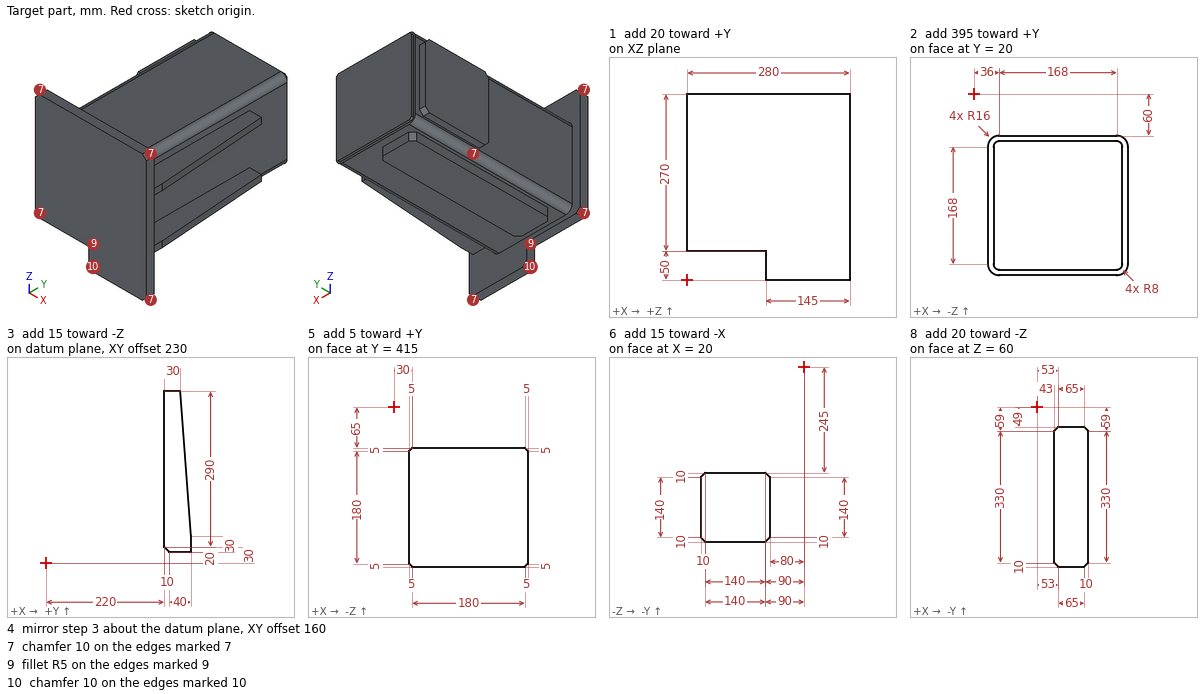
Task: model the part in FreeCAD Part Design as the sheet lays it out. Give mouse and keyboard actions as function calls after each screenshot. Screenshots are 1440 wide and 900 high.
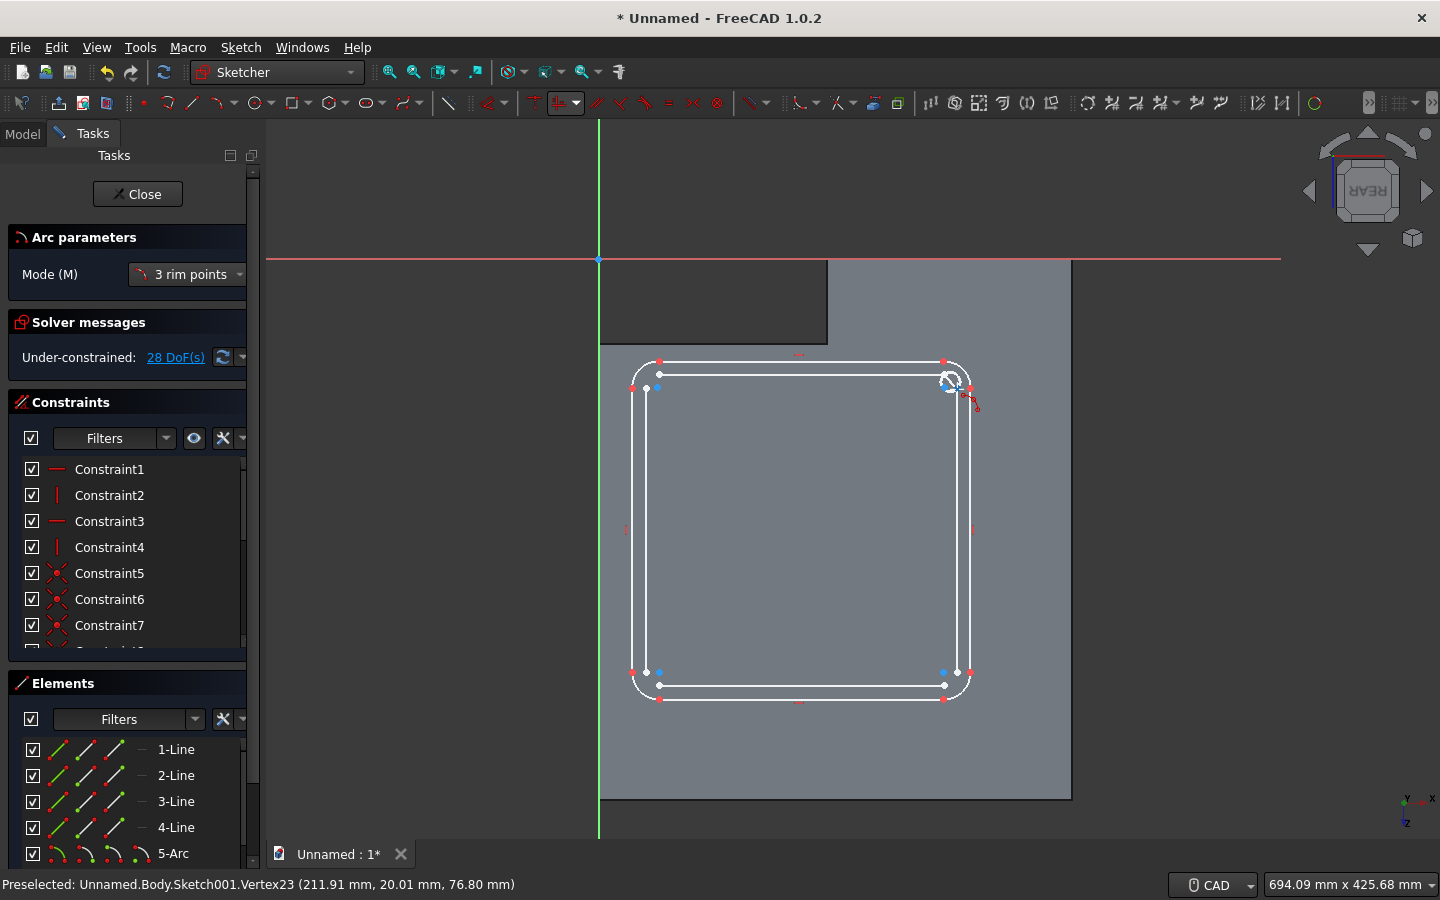
scroll(953, 378, up, 7)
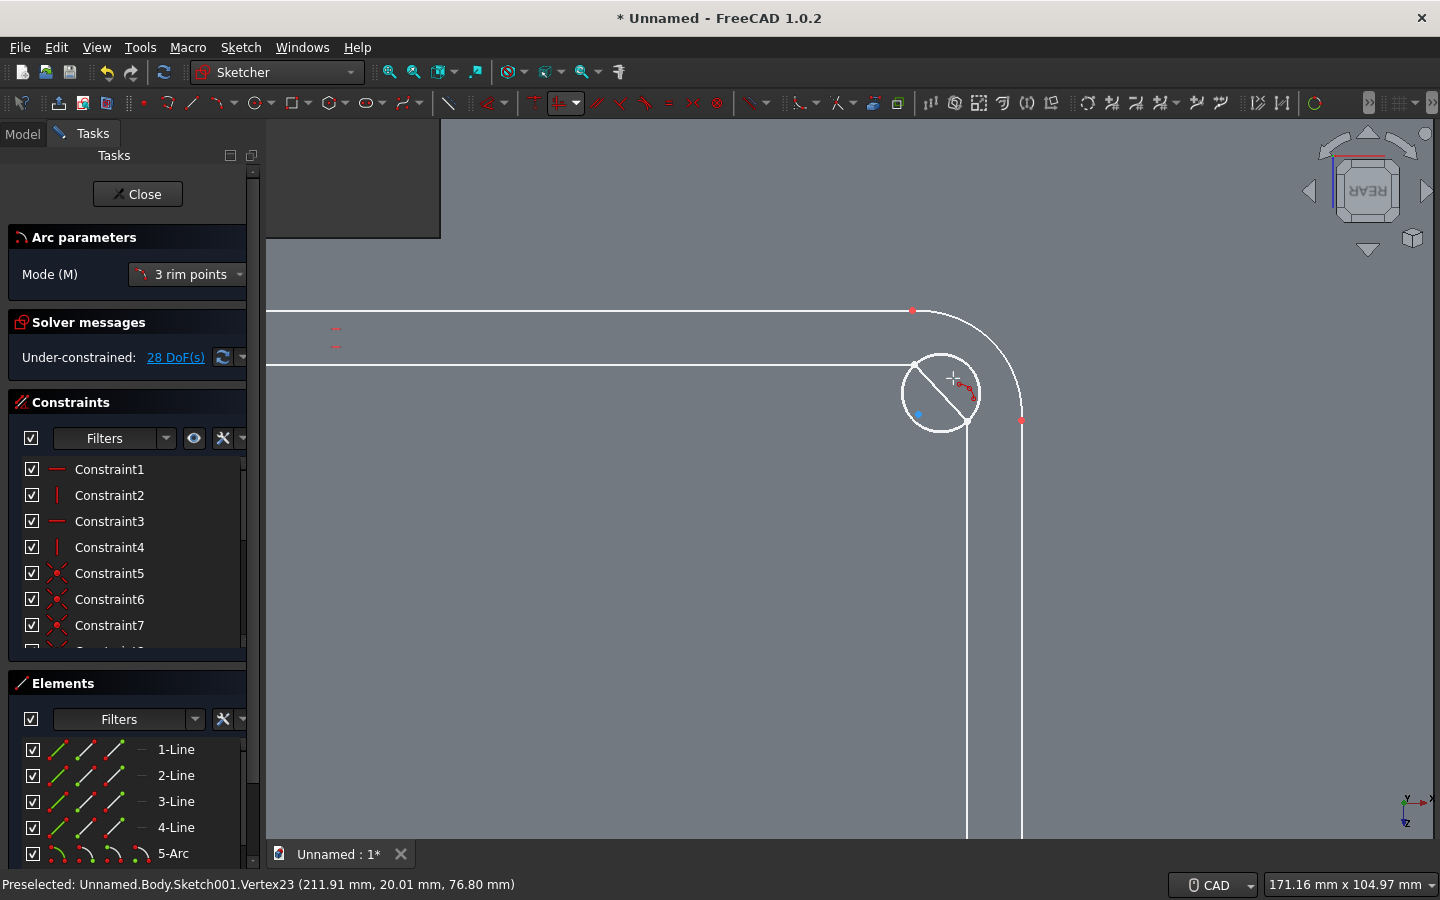
click(952, 377)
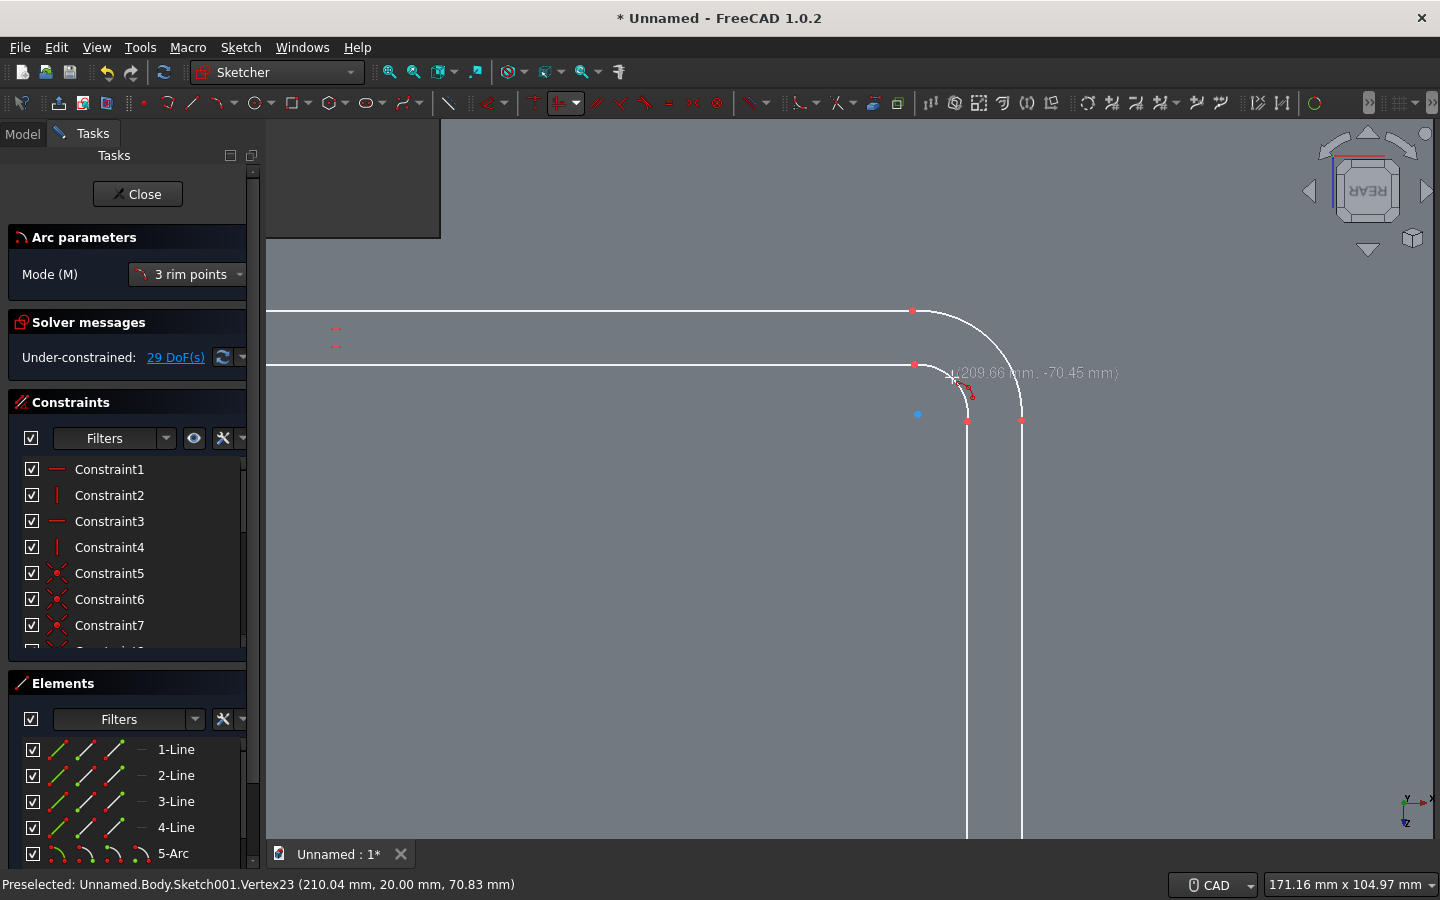
scroll(953, 378, down, 7)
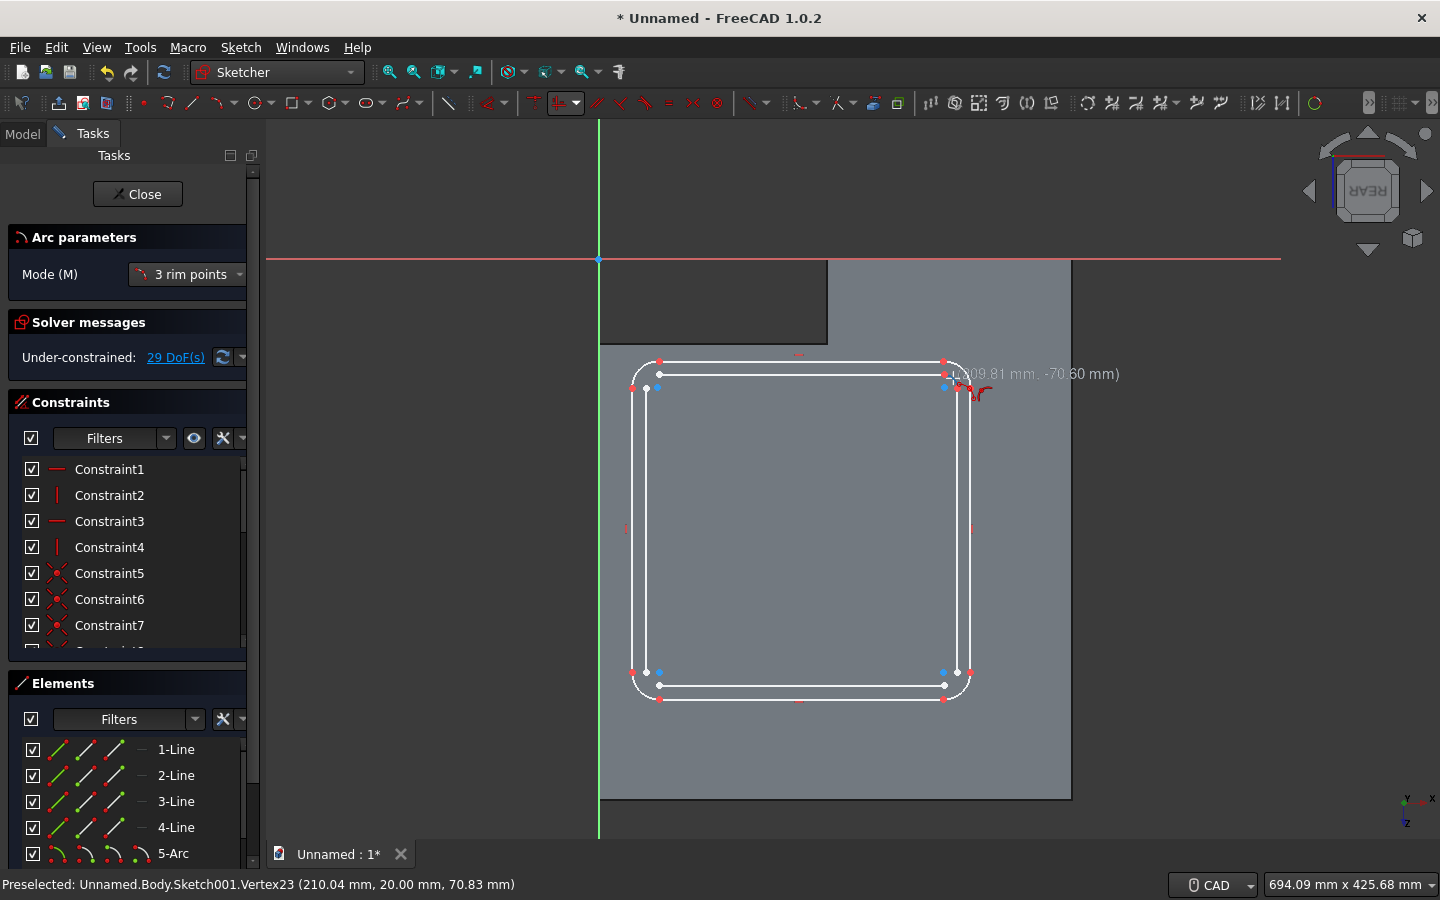
click(957, 673)
click(944, 686)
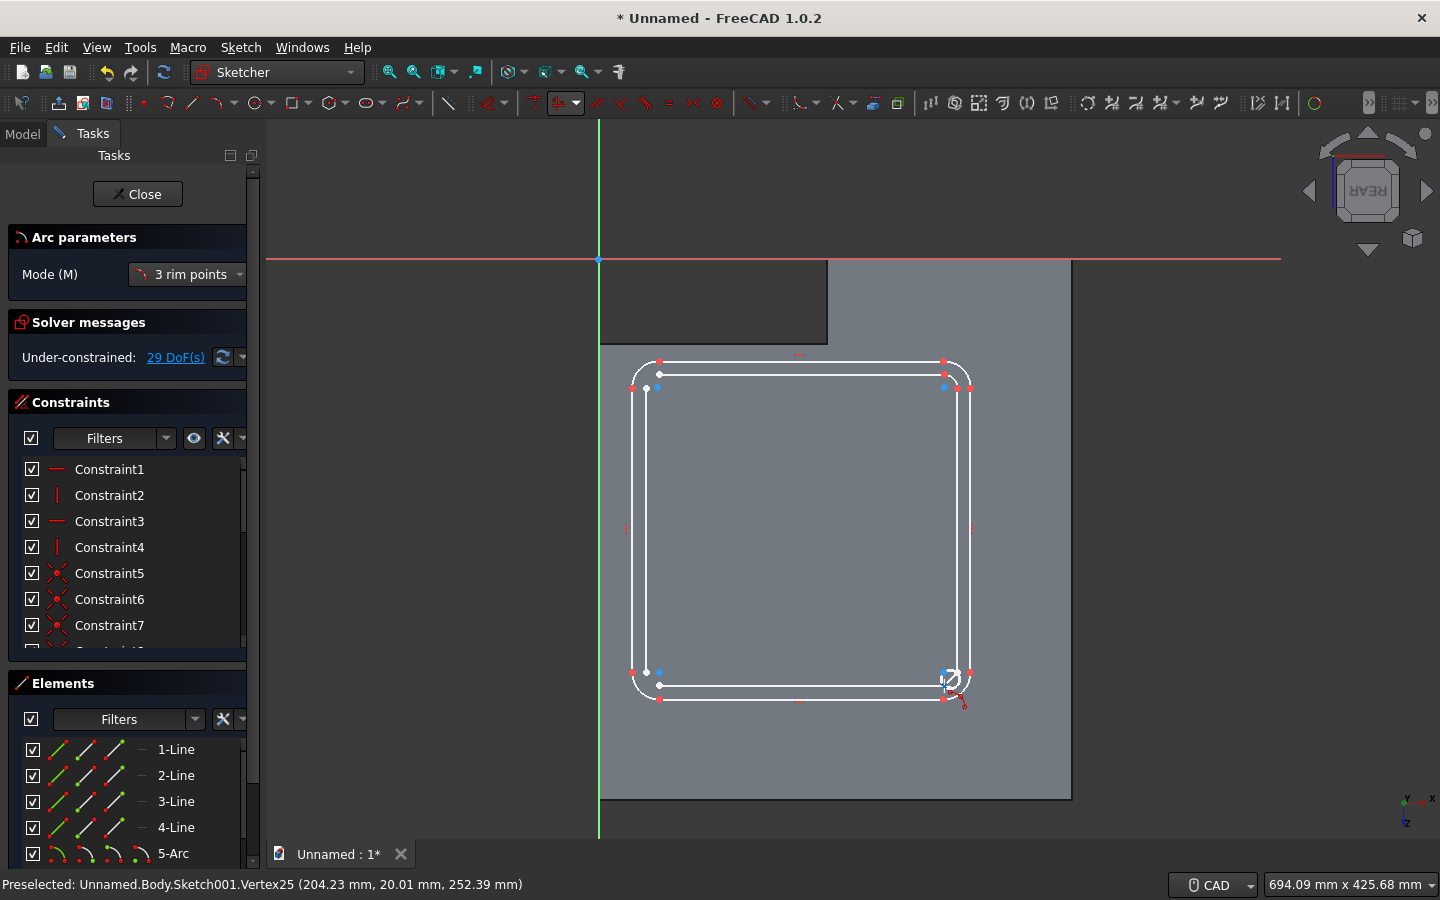
scroll(953, 681, up, 7)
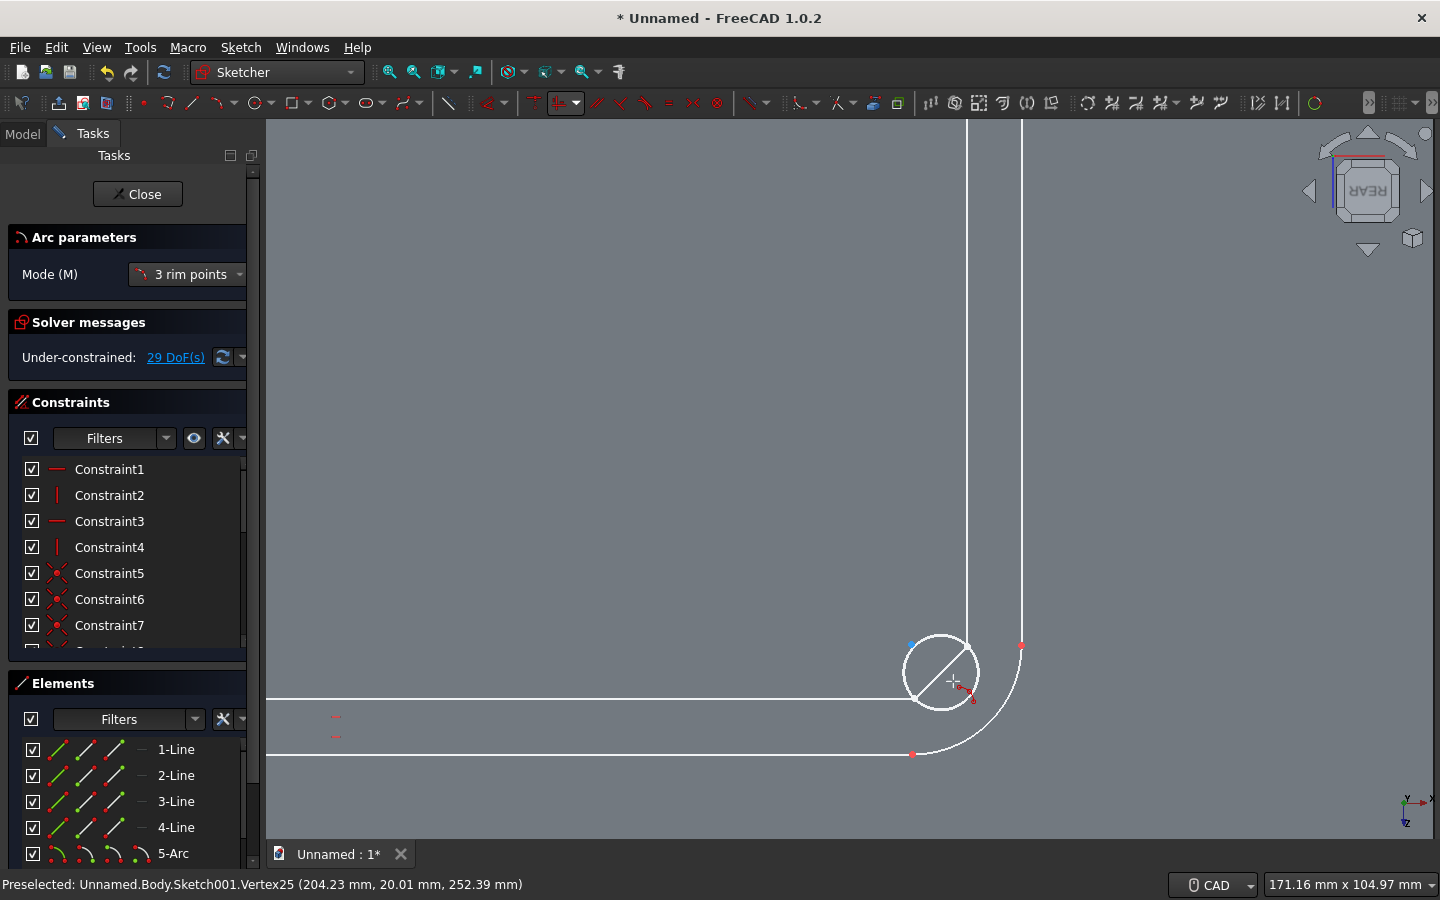
click(952, 680)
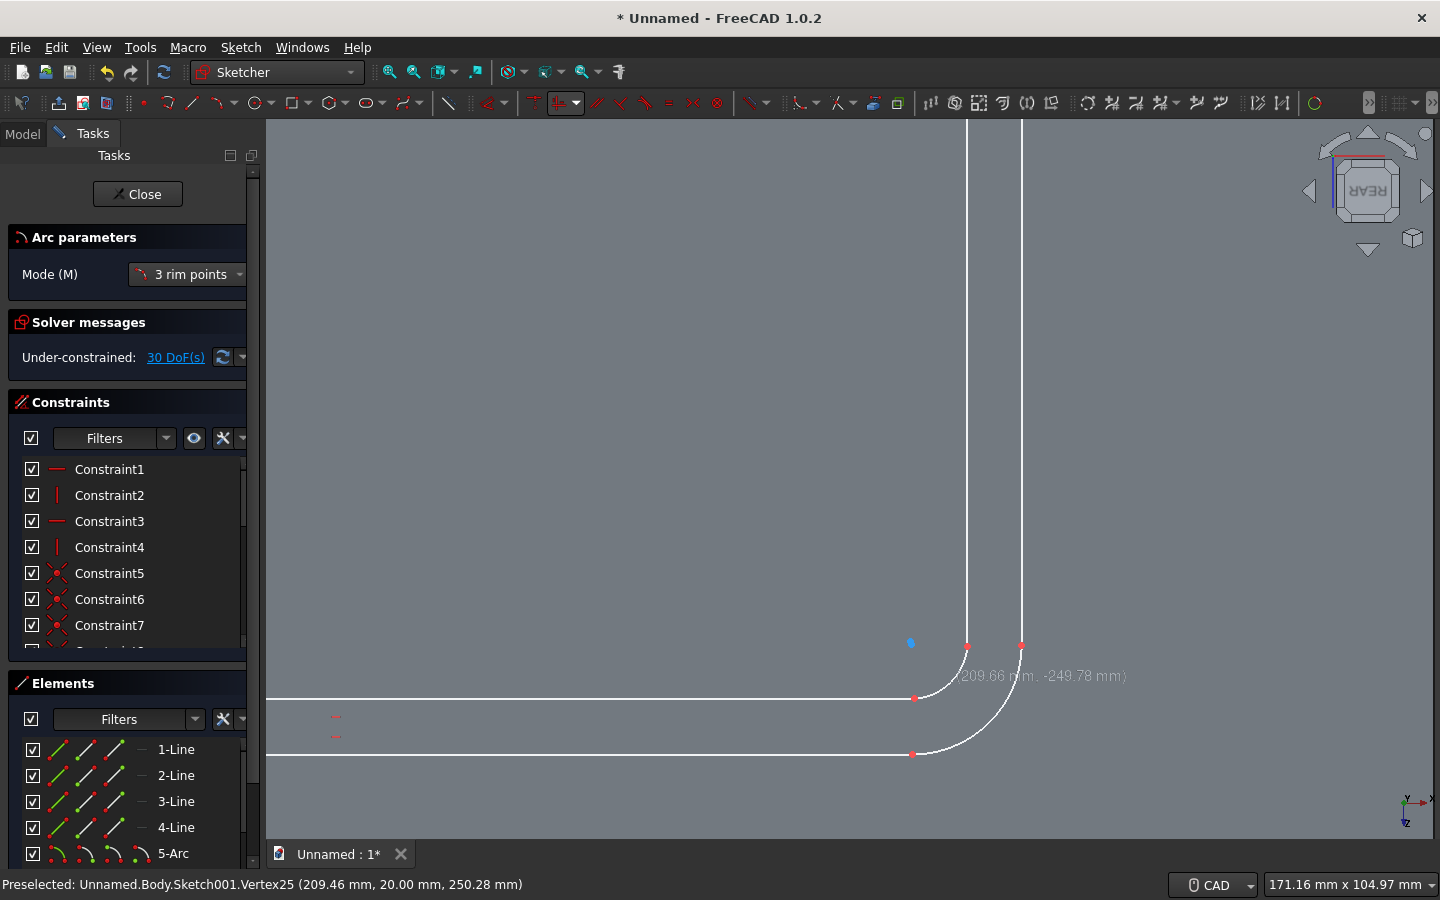
scroll(953, 682, down, 7)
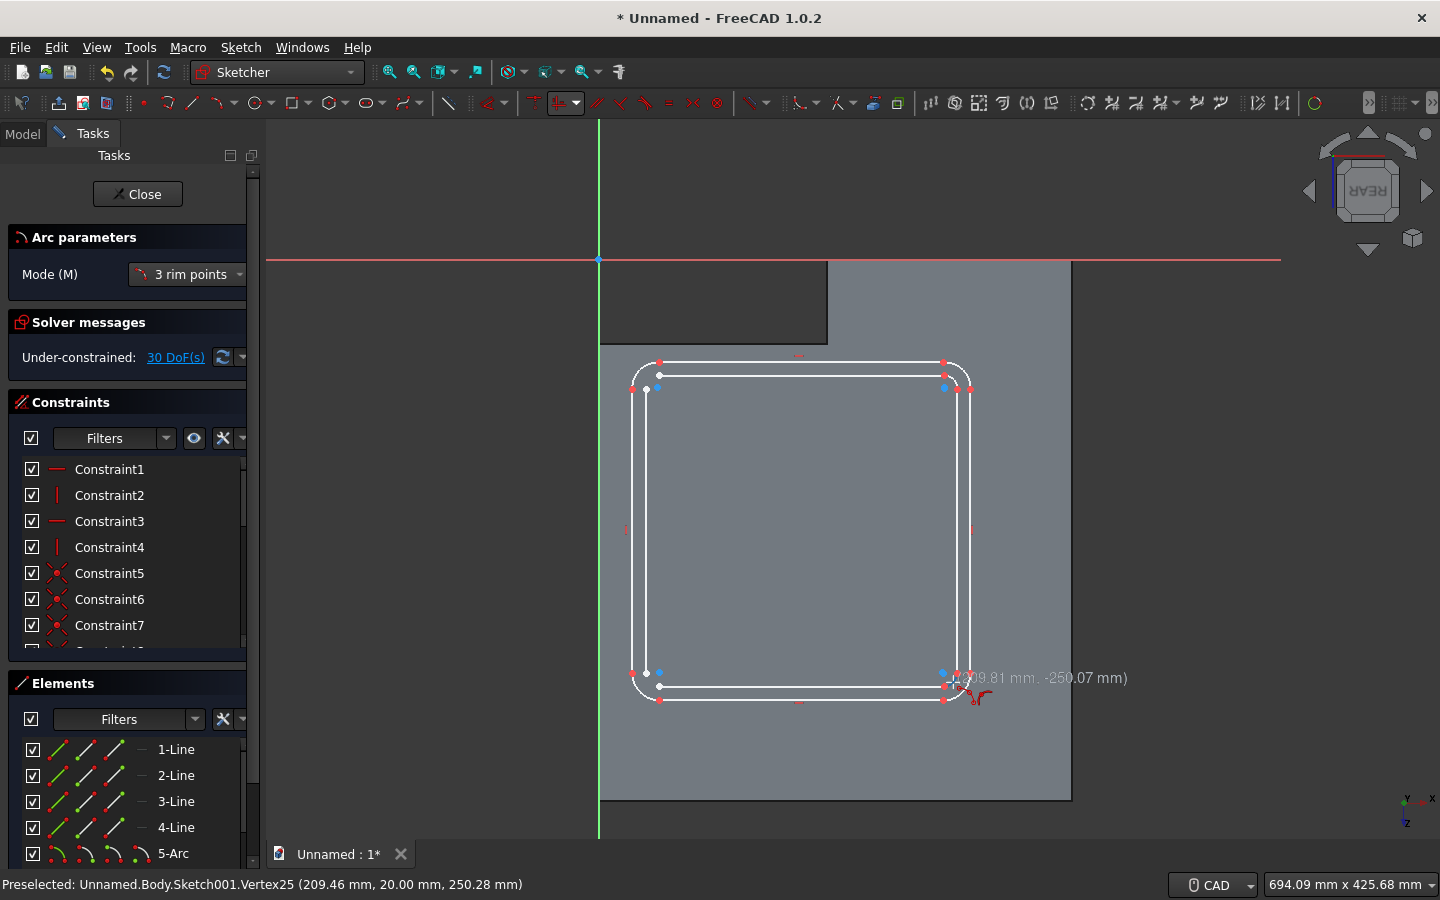
click(659, 687)
click(646, 674)